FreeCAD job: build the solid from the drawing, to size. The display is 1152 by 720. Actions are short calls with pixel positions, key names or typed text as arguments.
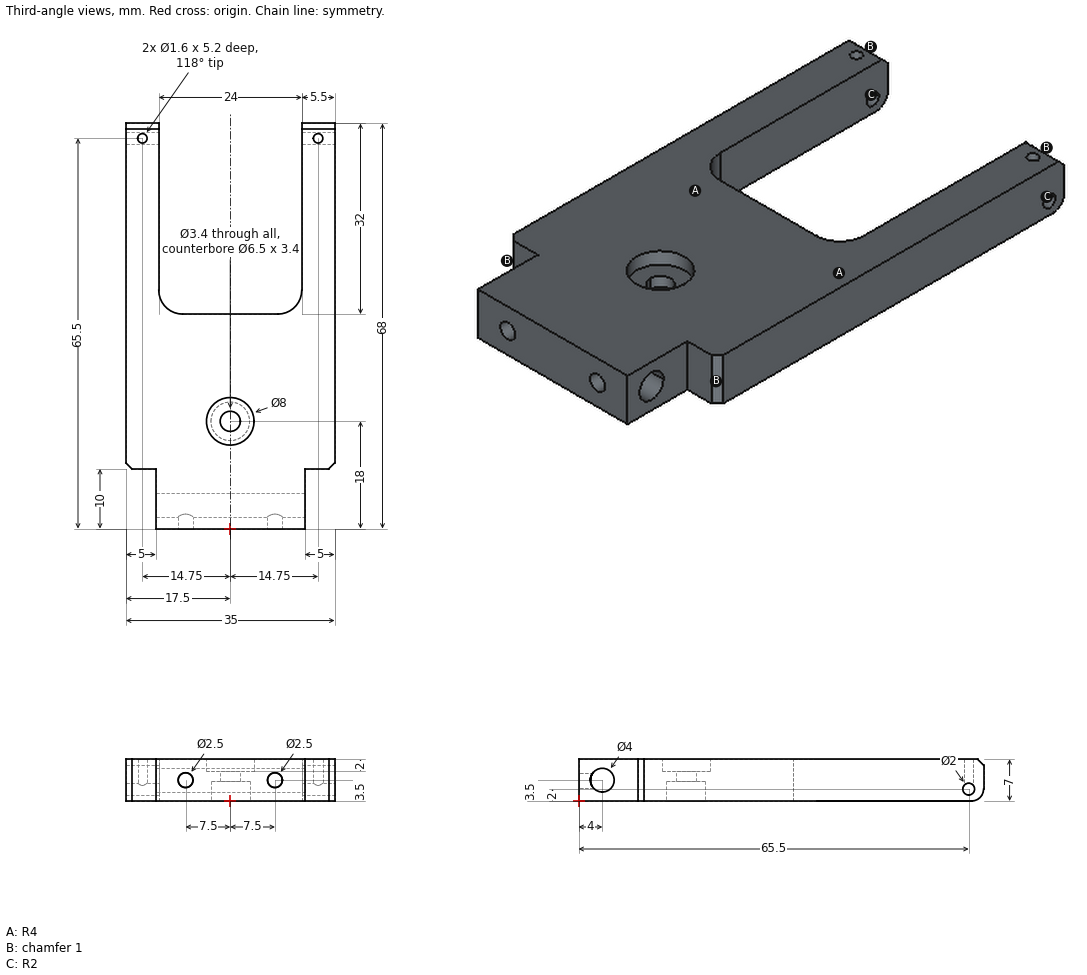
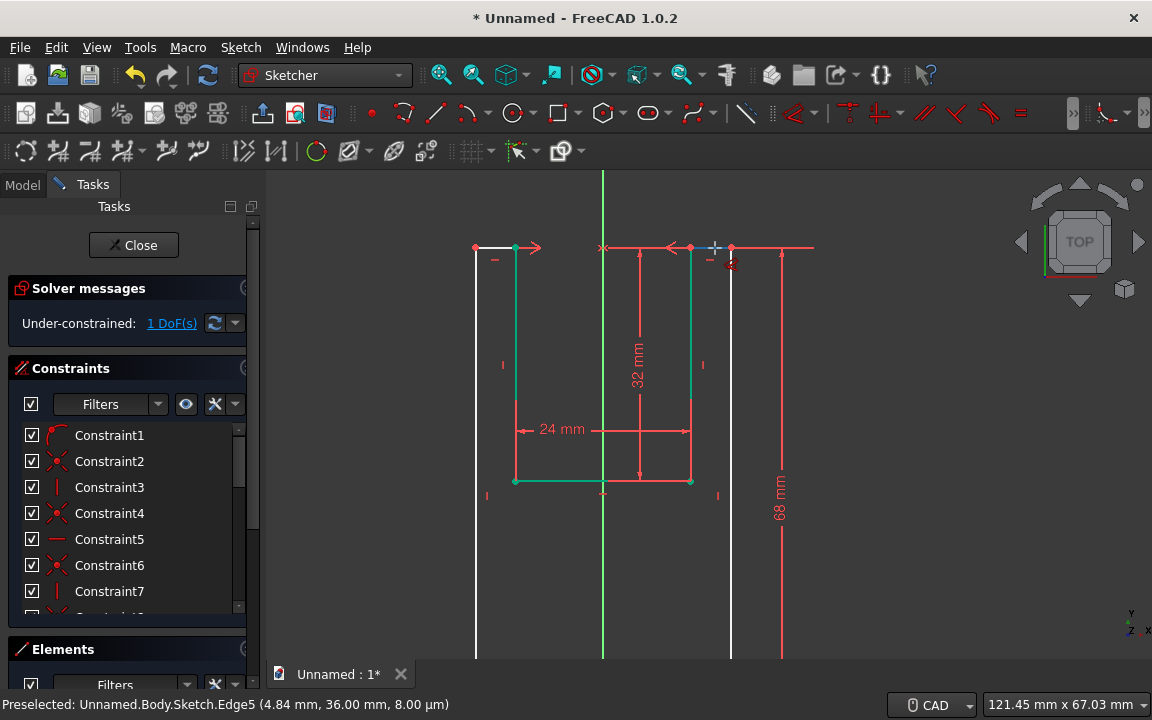
click(715, 248)
click(711, 214)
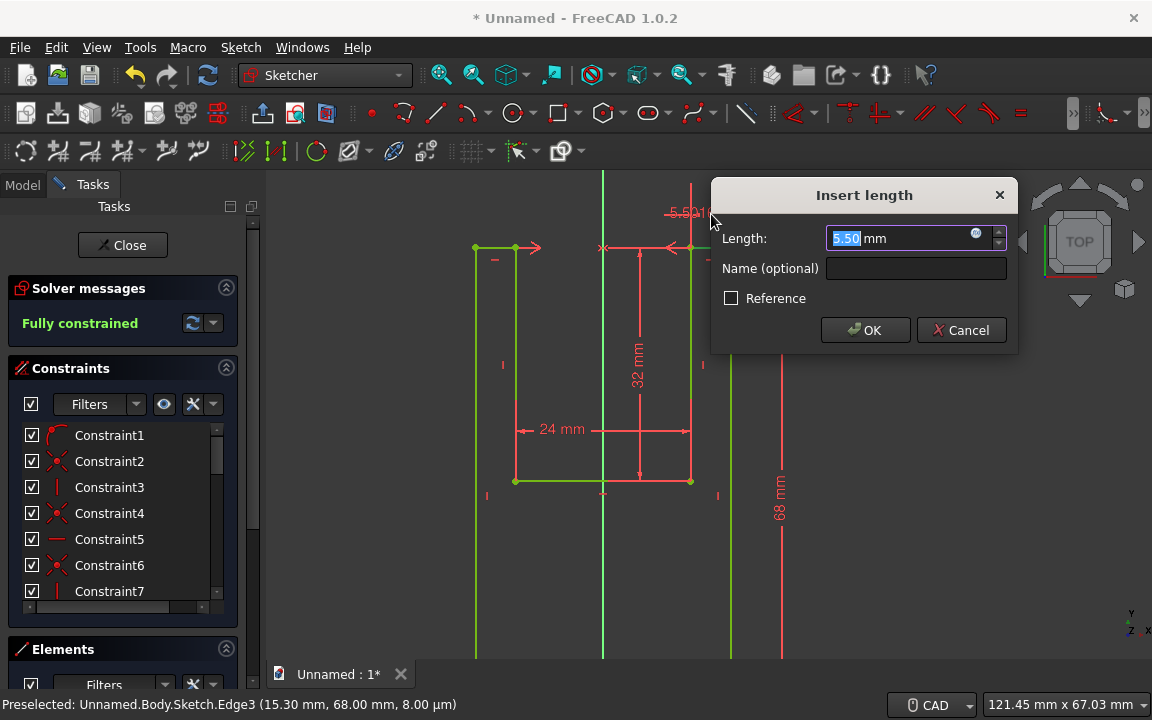
text(5.5)
key(Return)
key(Escape)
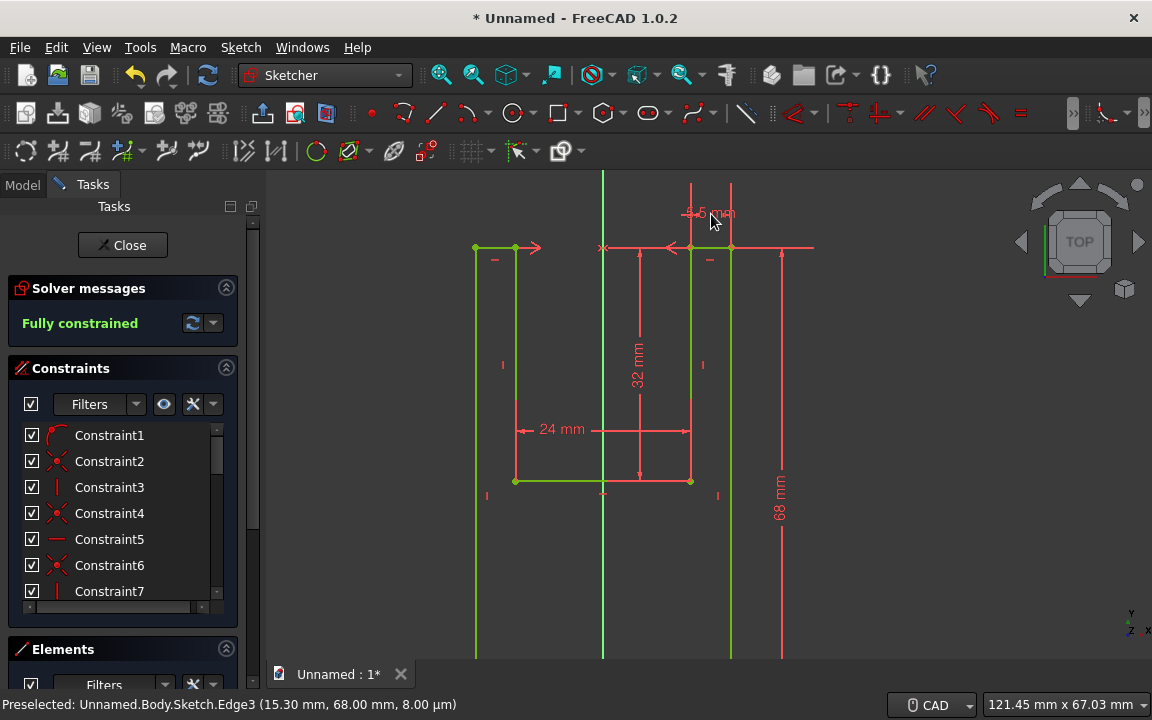
click(123, 245)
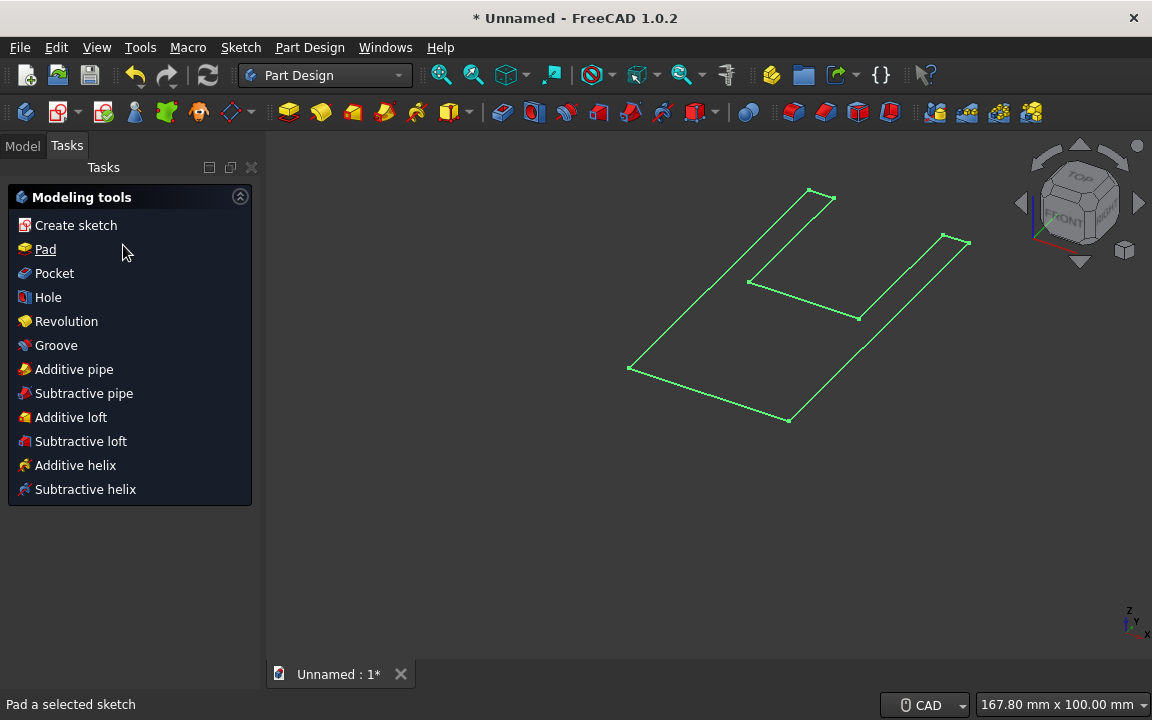
click(290, 112)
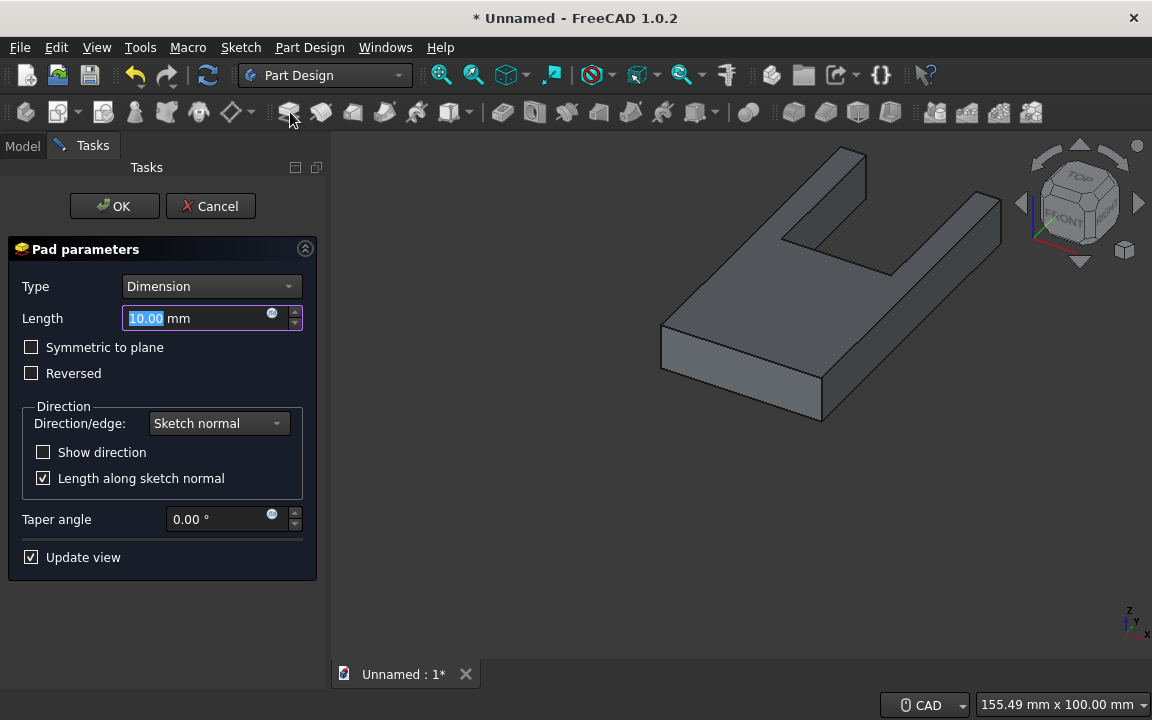
text(7)
key(Tab)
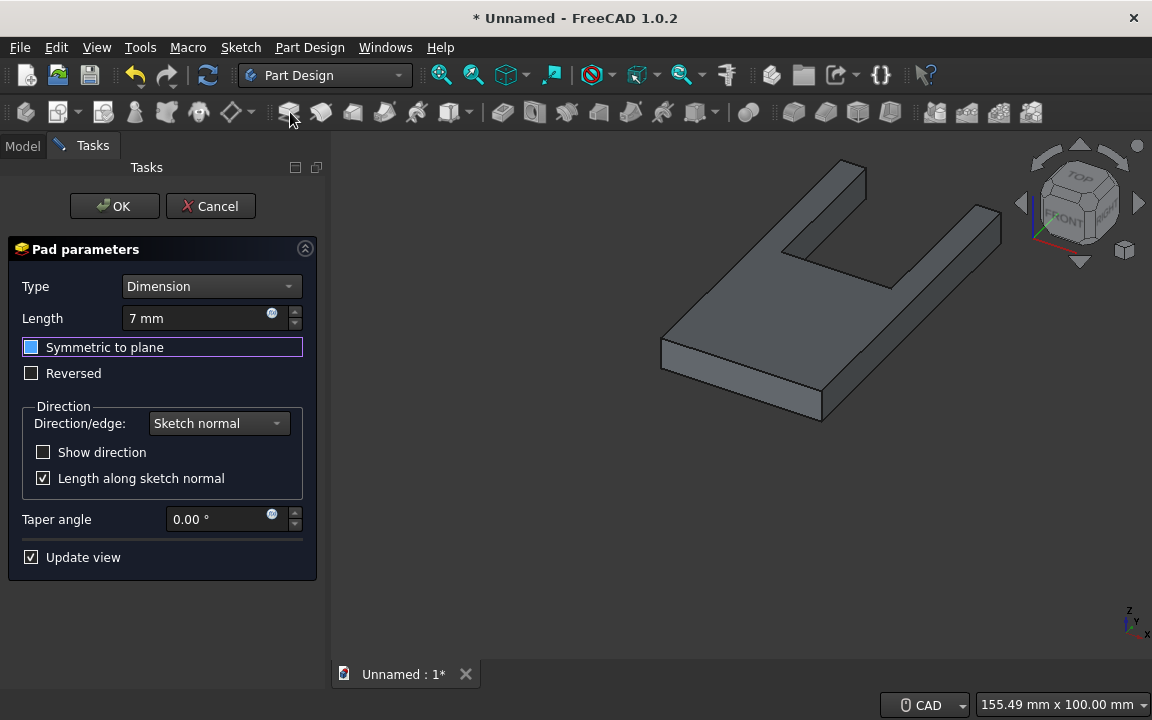
click(115, 206)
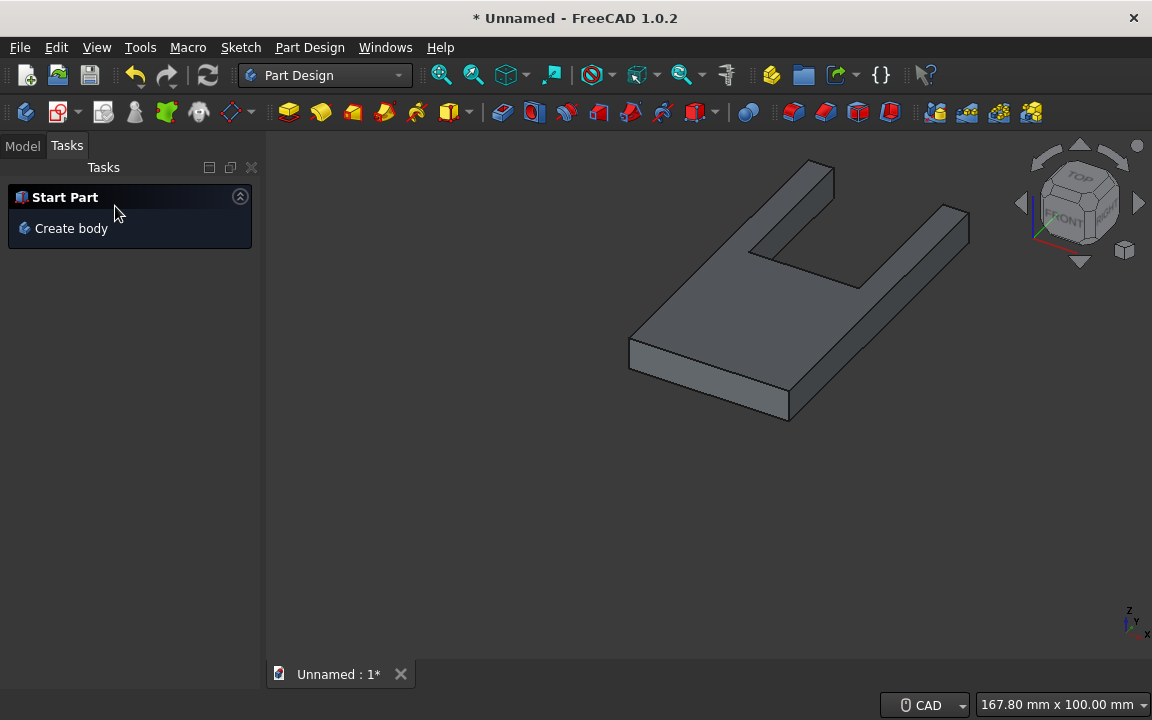
click(956, 240)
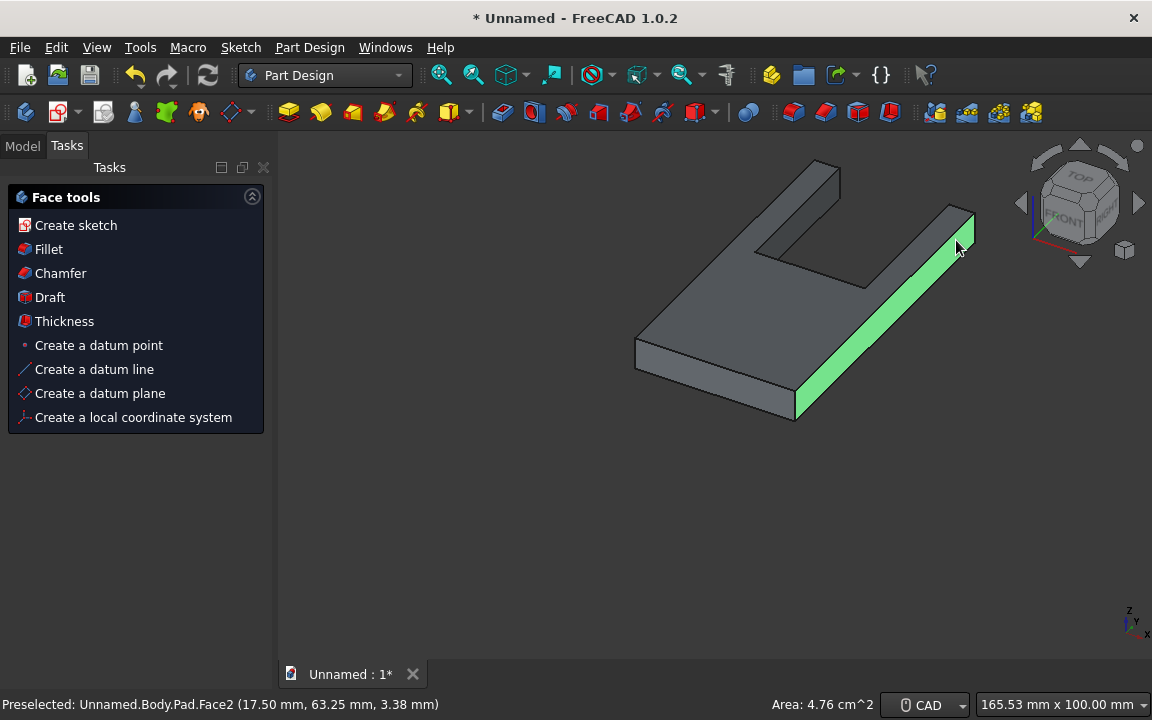
click(58, 112)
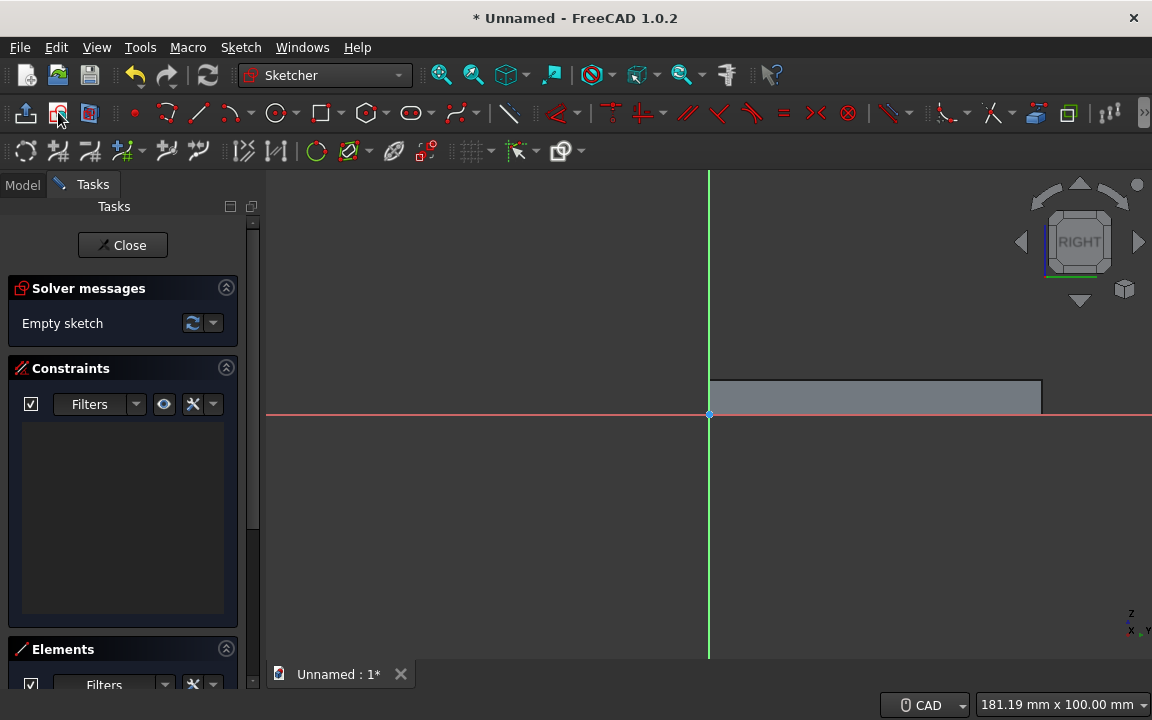
scroll(640, 414, down, 5)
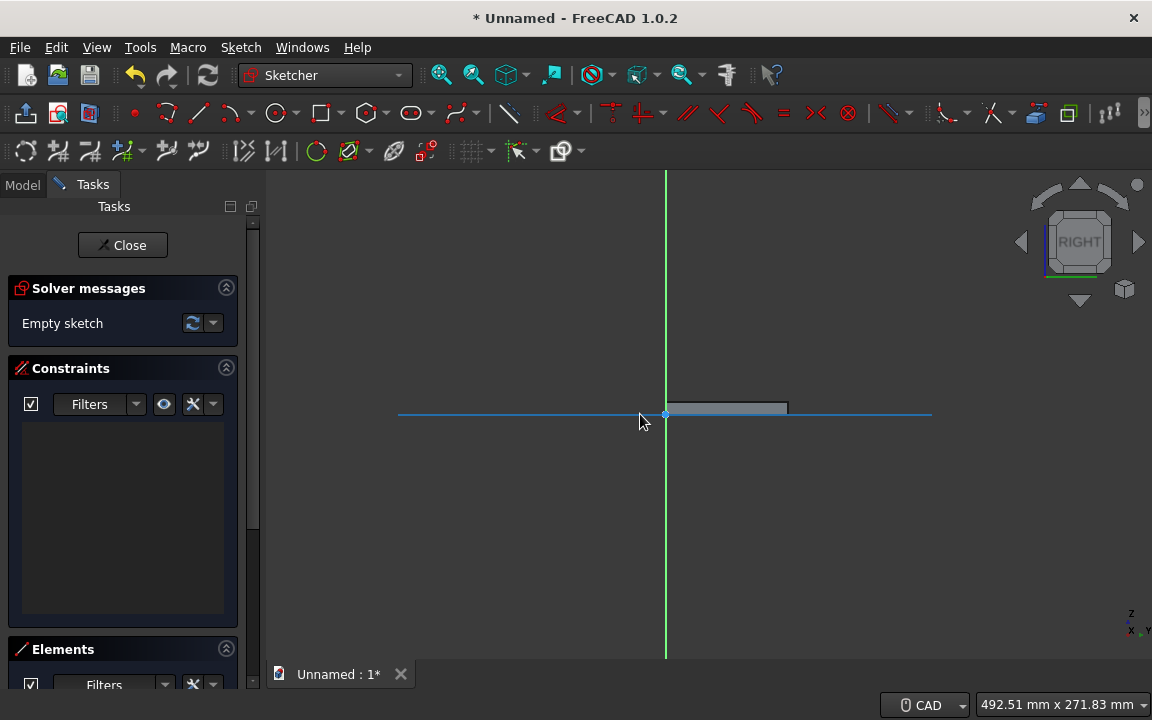
scroll(791, 411, up, 15)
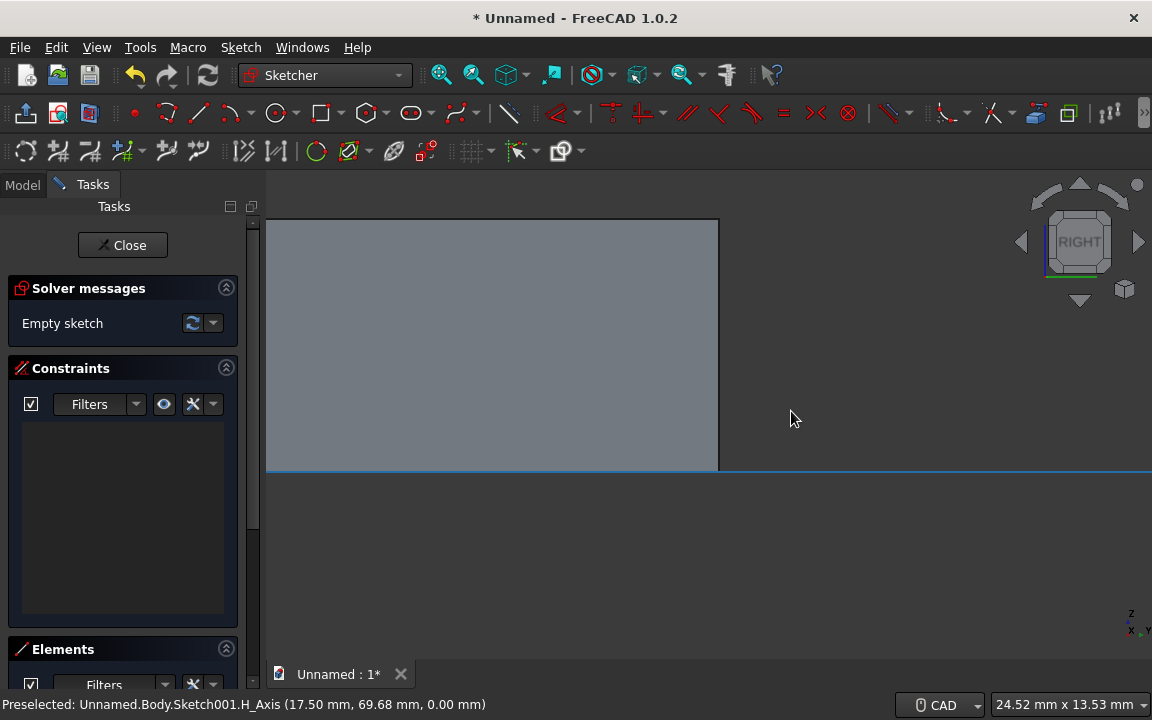
scroll(625, 395, up, 7)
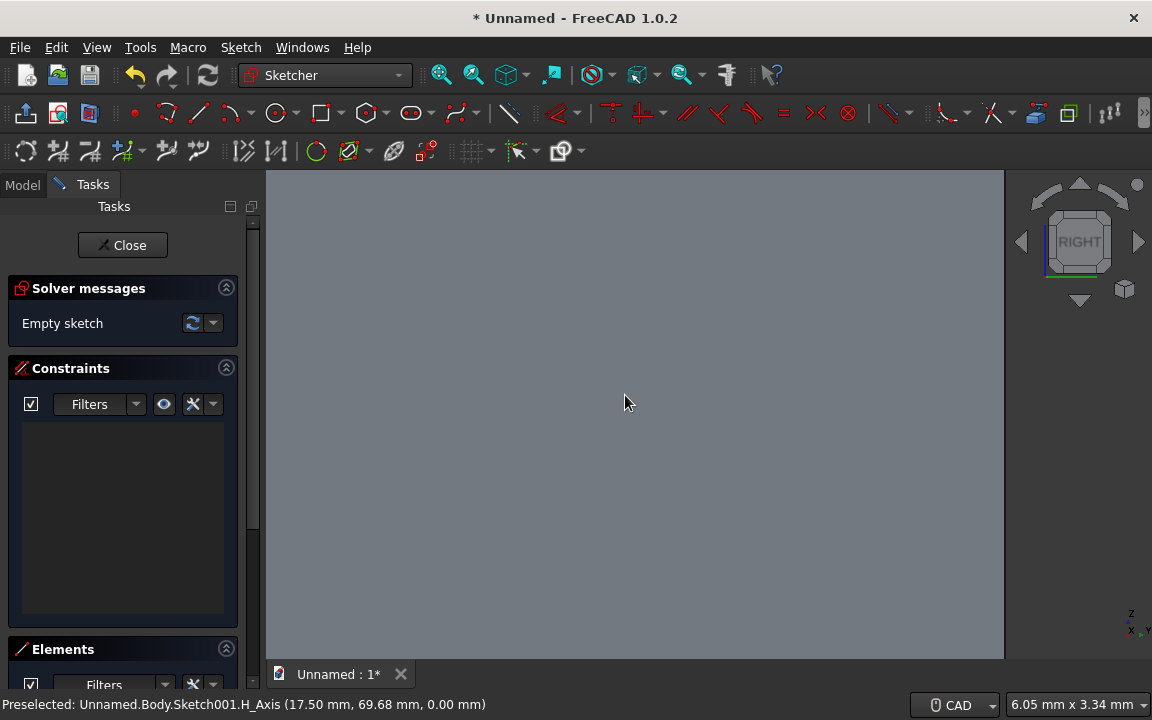
key(g)
key(c)